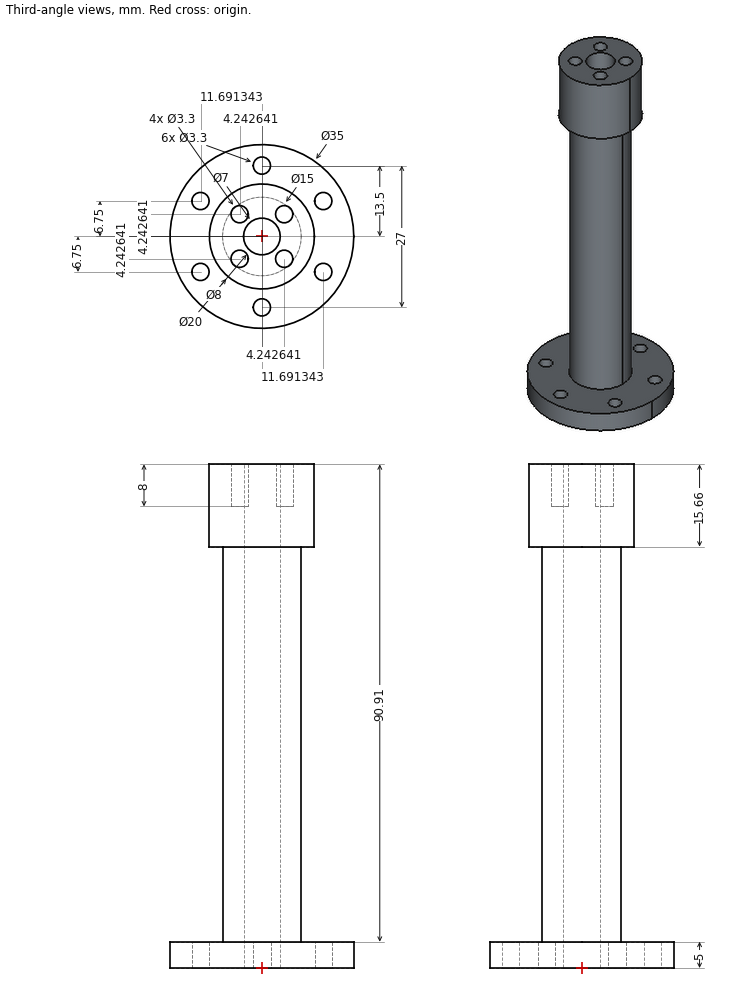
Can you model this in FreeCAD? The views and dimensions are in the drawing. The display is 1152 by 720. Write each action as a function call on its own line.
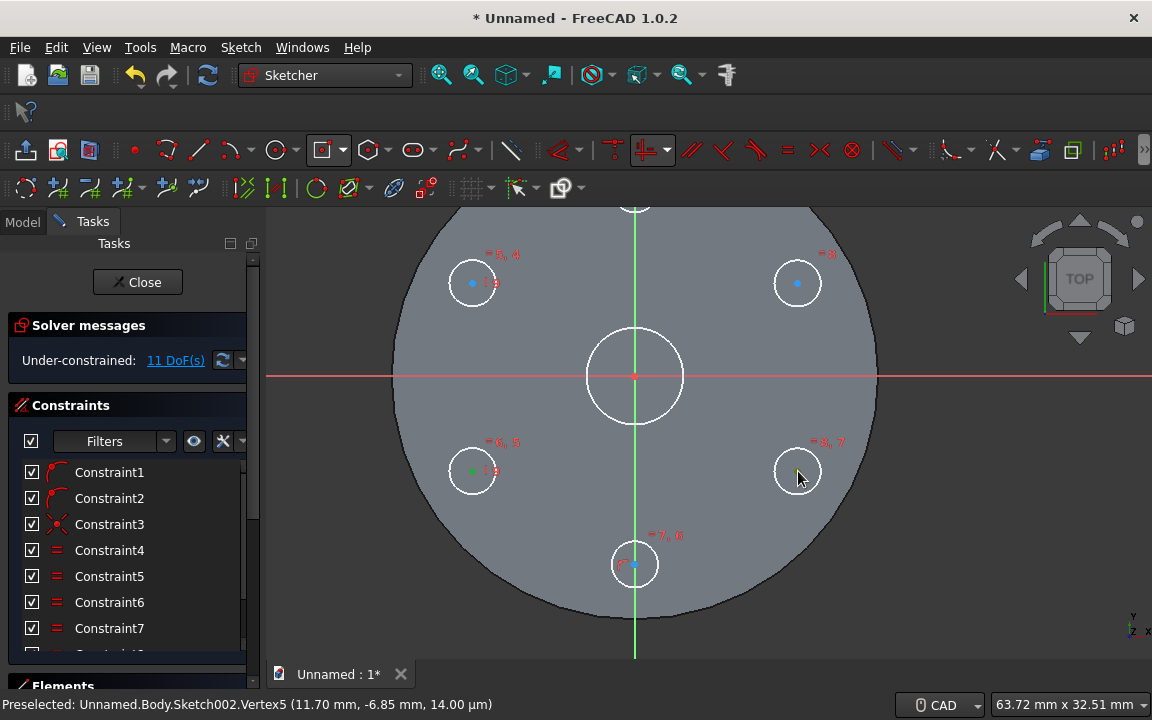
key(h)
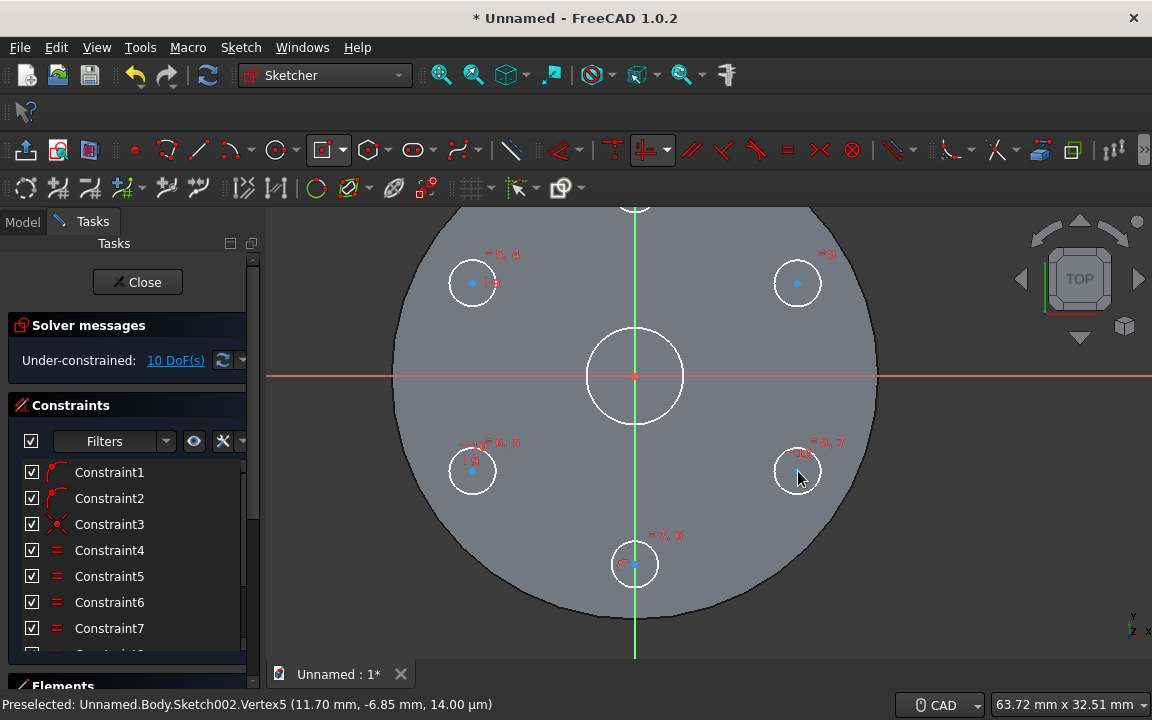
click(798, 471)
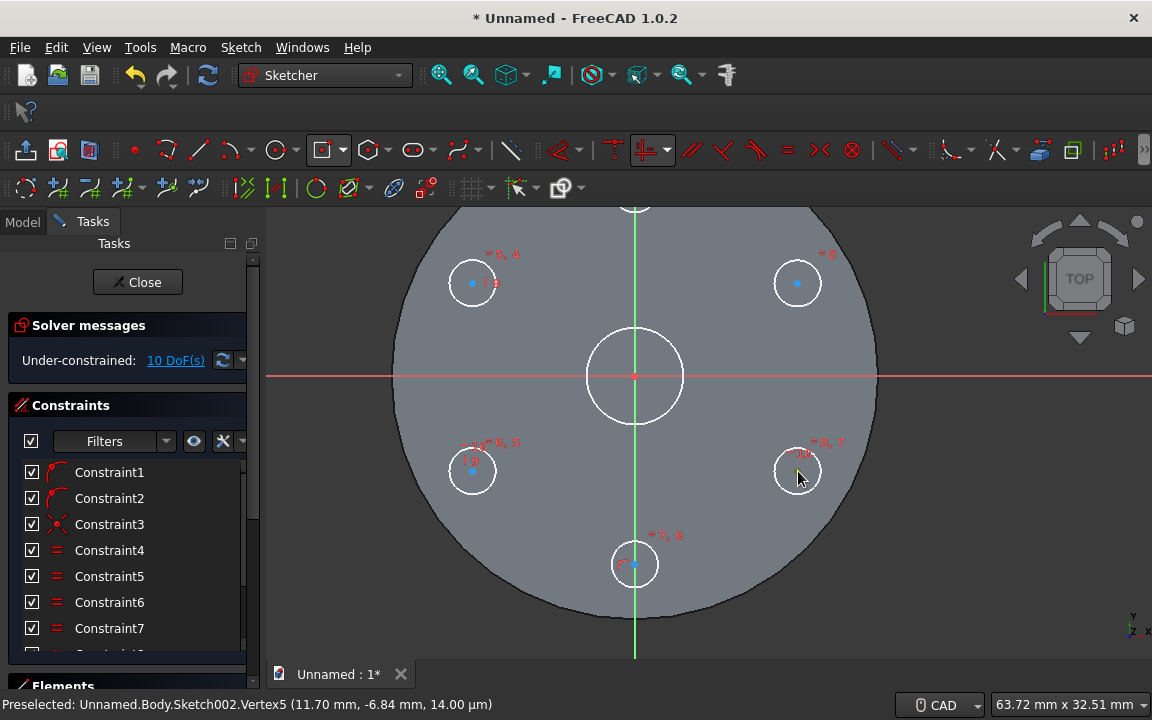
click(798, 283)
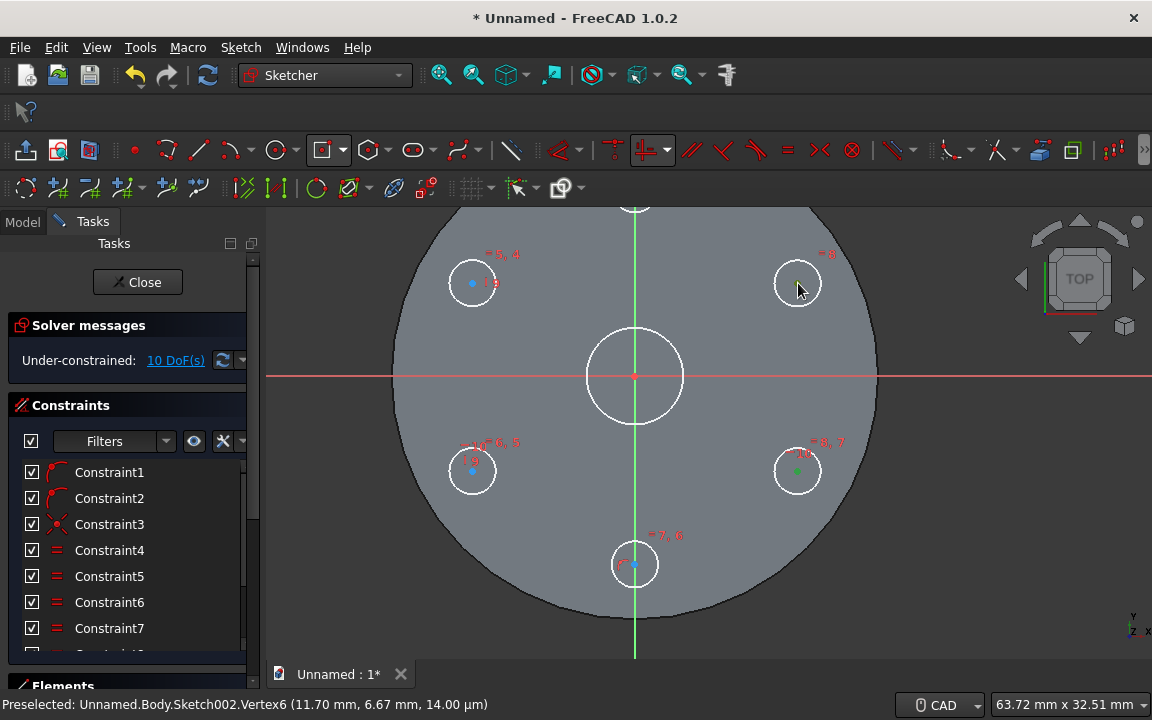
key(v)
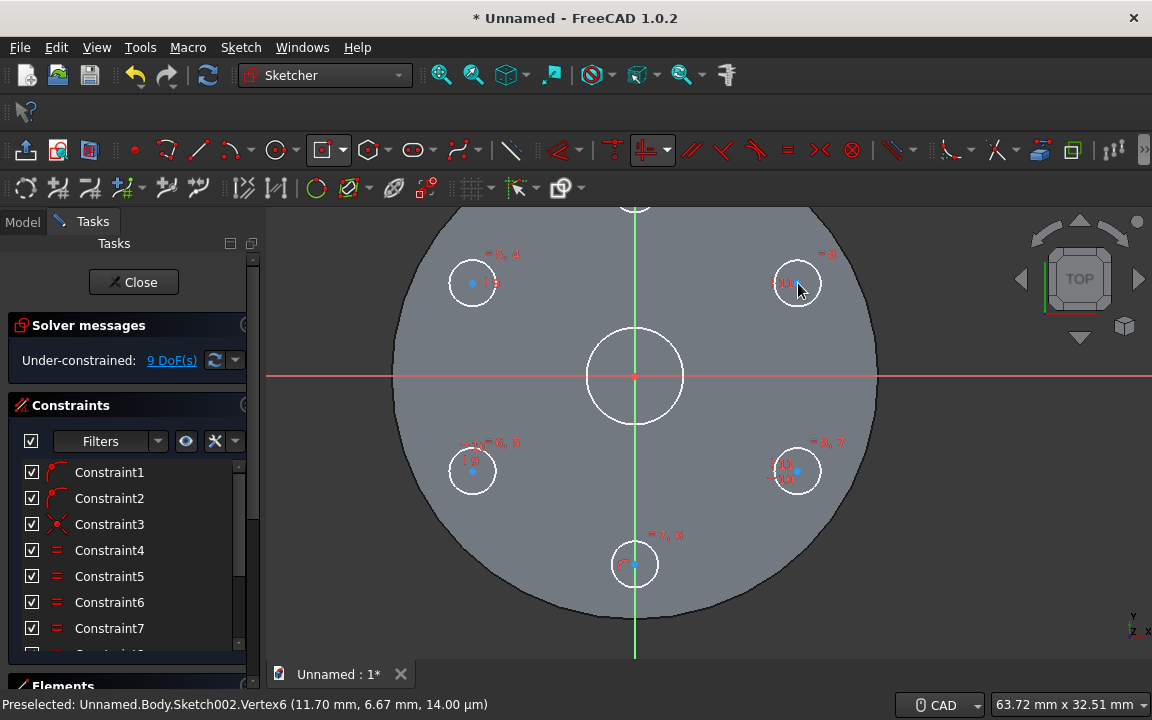
click(473, 283)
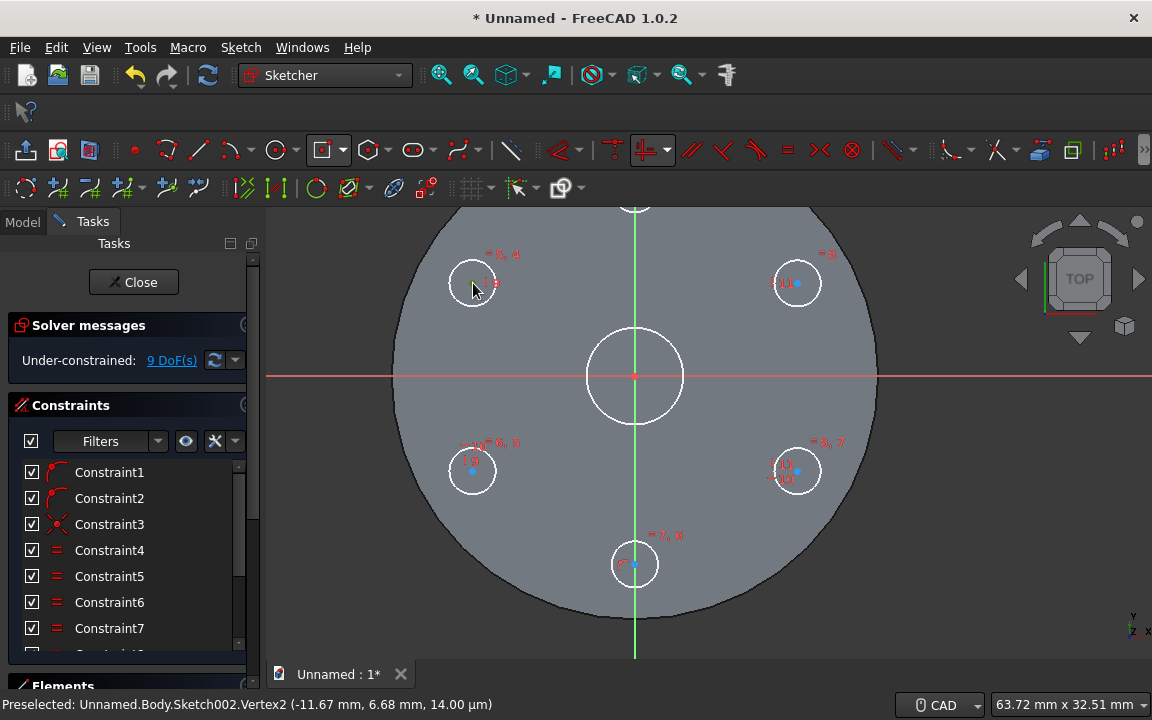
click(798, 283)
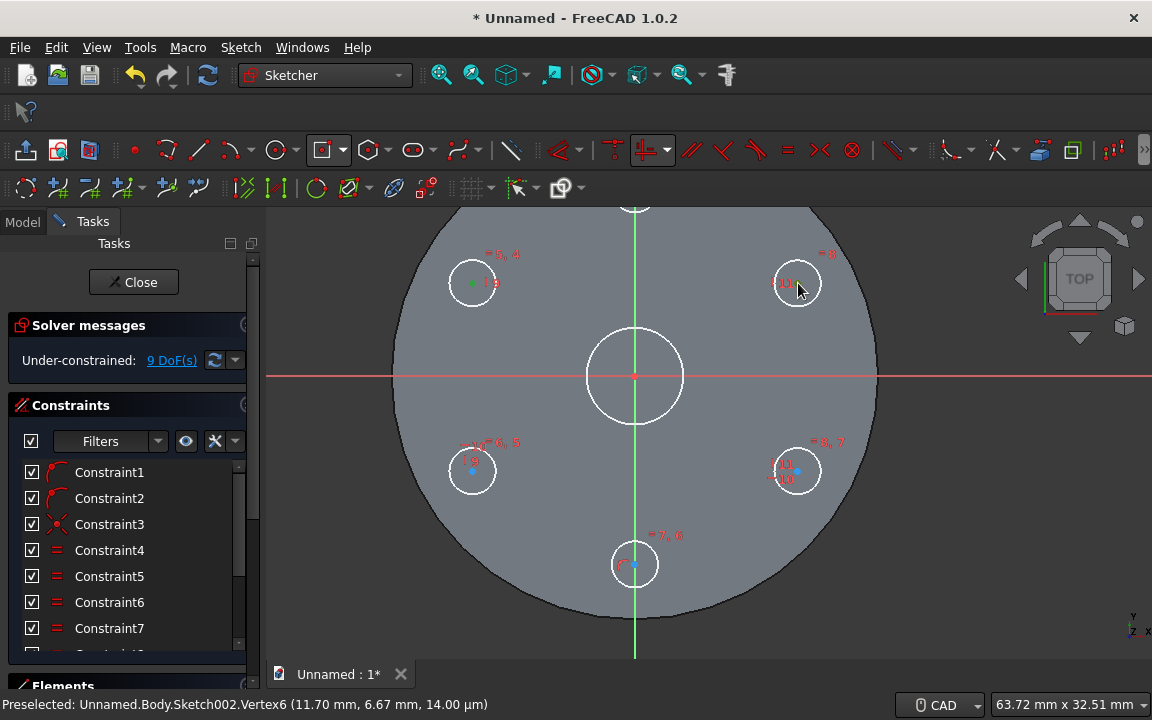
key(h)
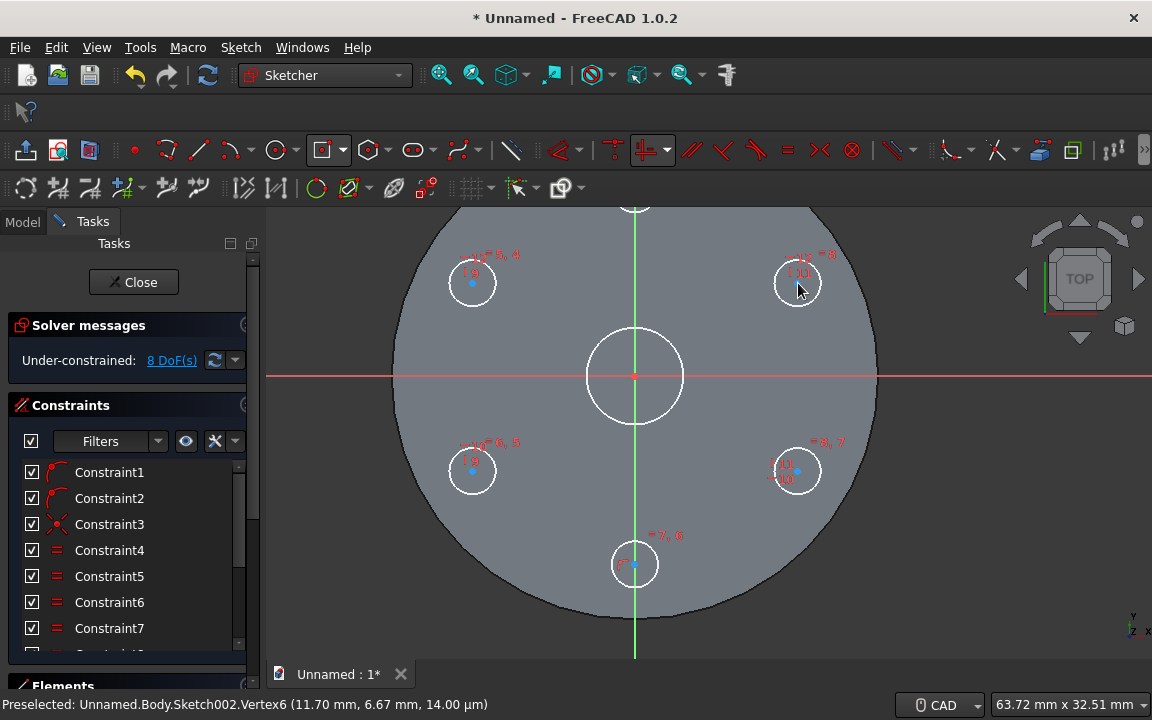
key(d)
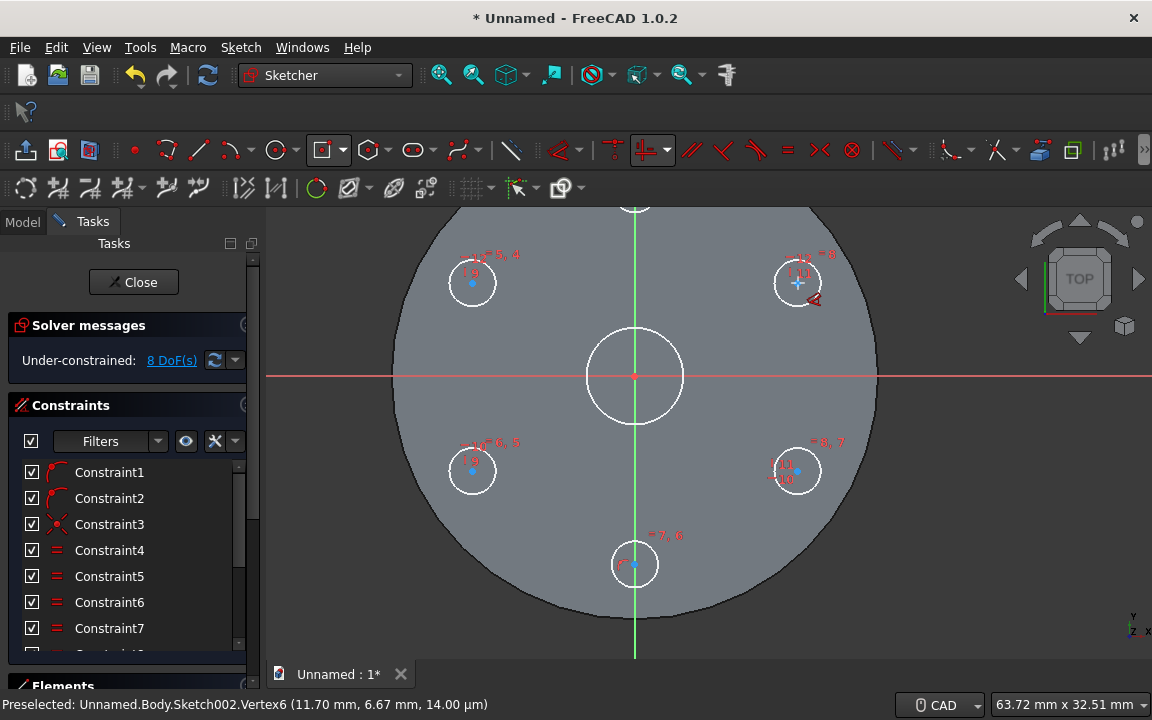
scroll(652, 549, down, 2)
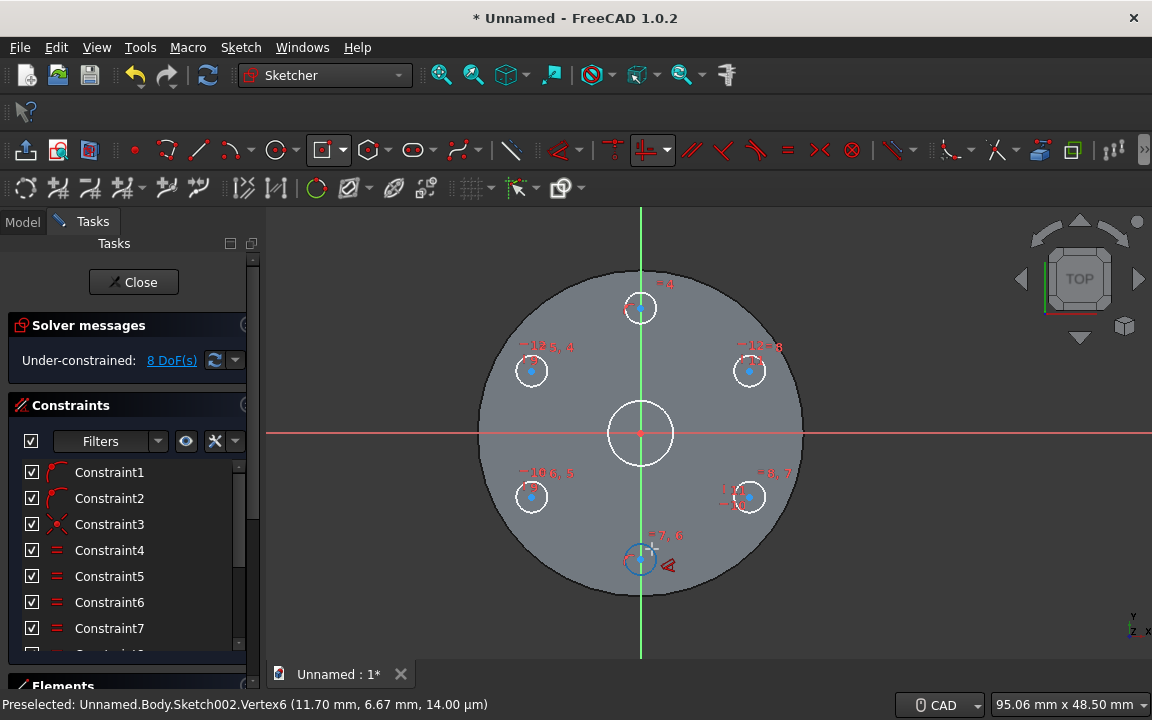
scroll(652, 297, up, 2)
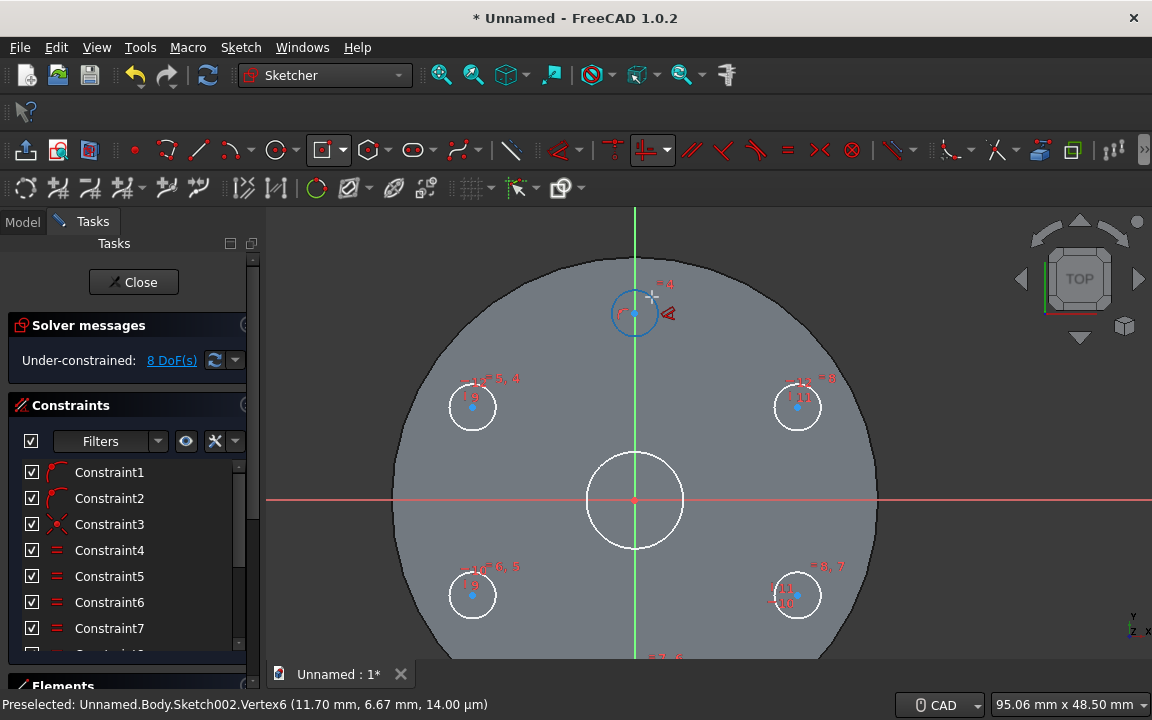
click(651, 297)
click(673, 274)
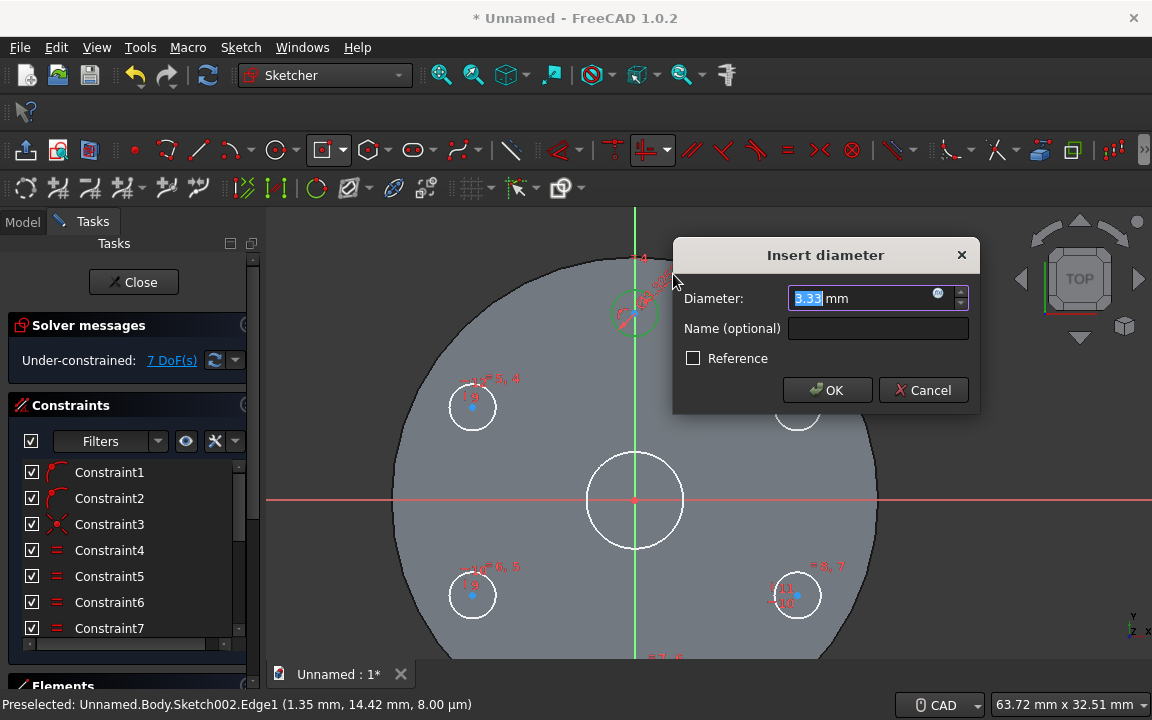
text(3.3)
key(Return)